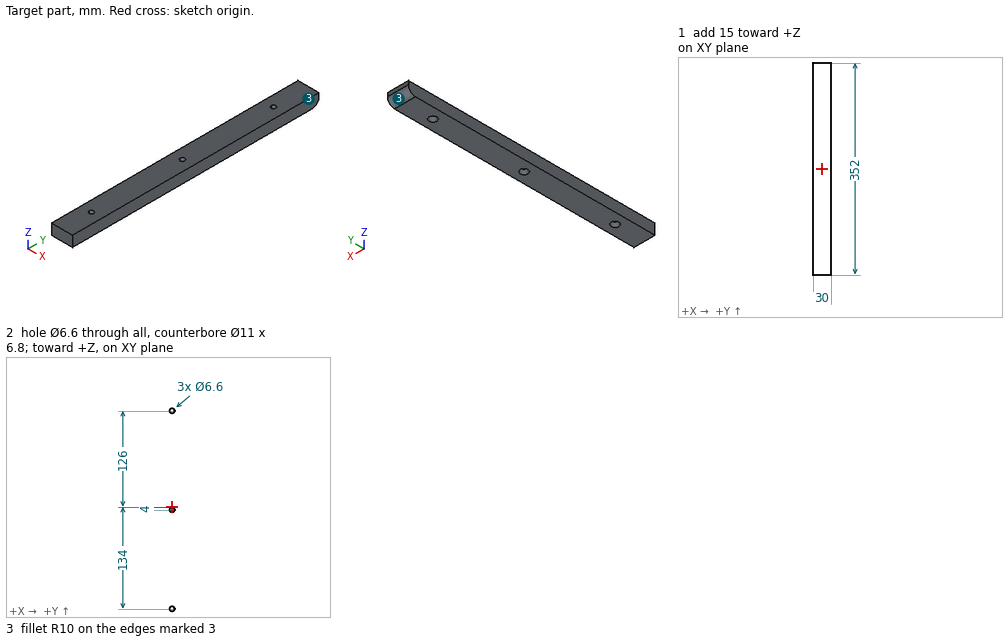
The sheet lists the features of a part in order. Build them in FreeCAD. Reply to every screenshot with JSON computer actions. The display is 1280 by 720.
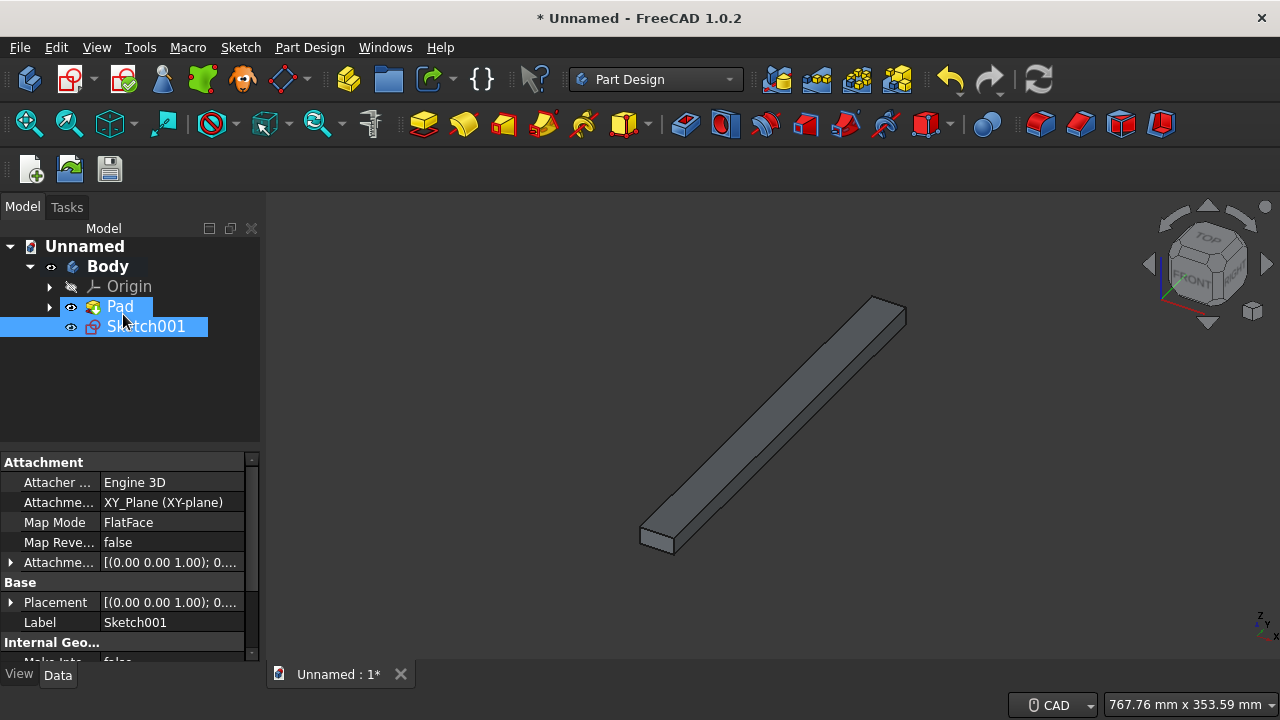
{"action": "left_click", "coordinate": [726, 124]}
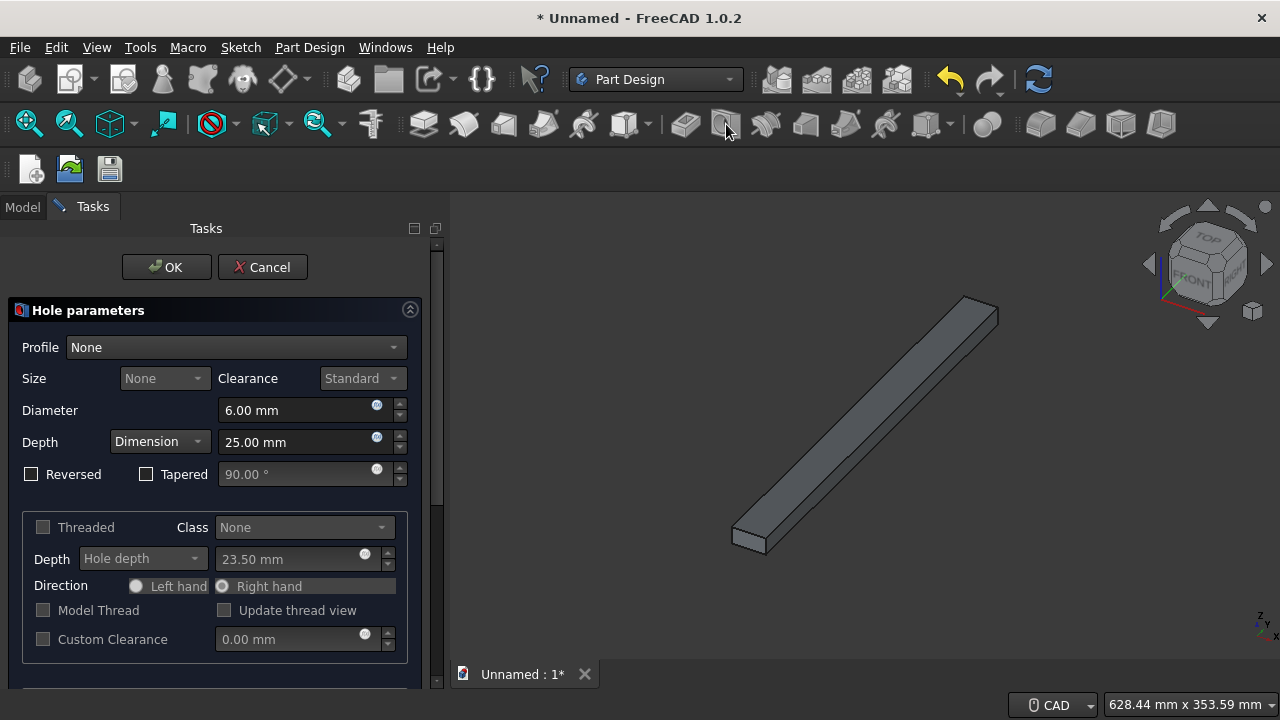
{"action": "triple_click", "coordinate": [305, 410]}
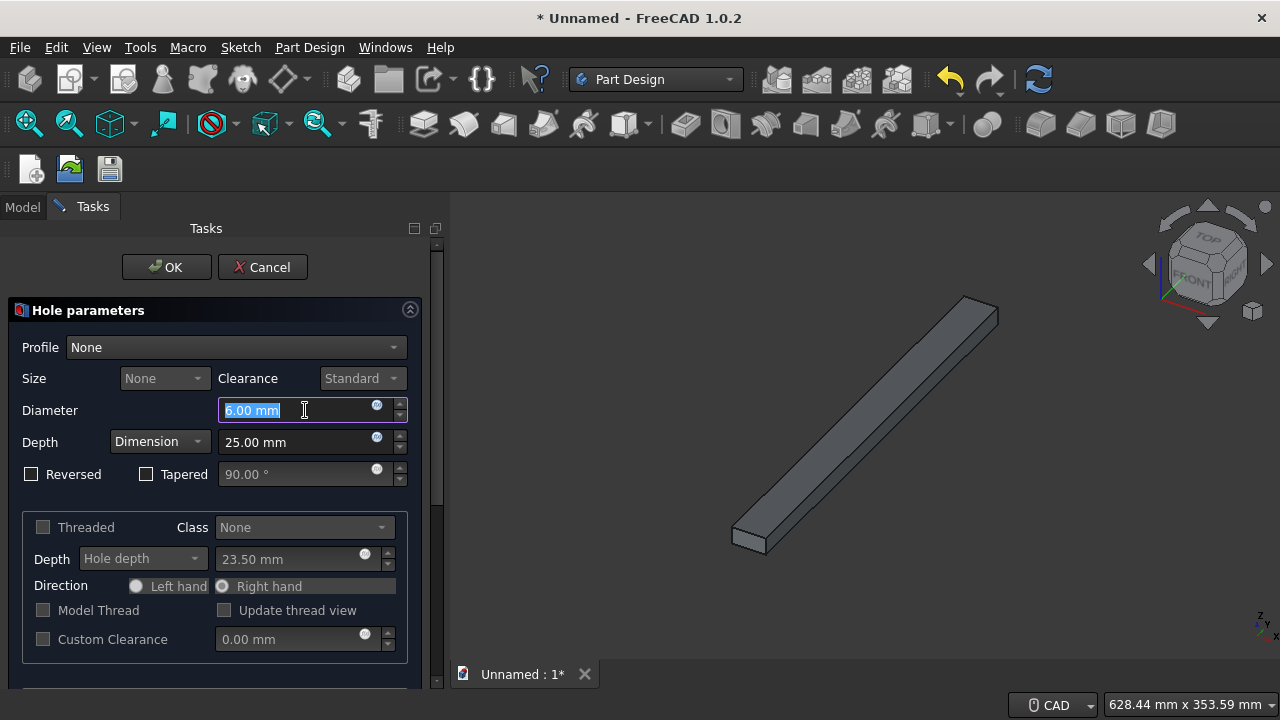
{"action": "type", "text": "6.6"}
{"action": "key", "text": "Tab"}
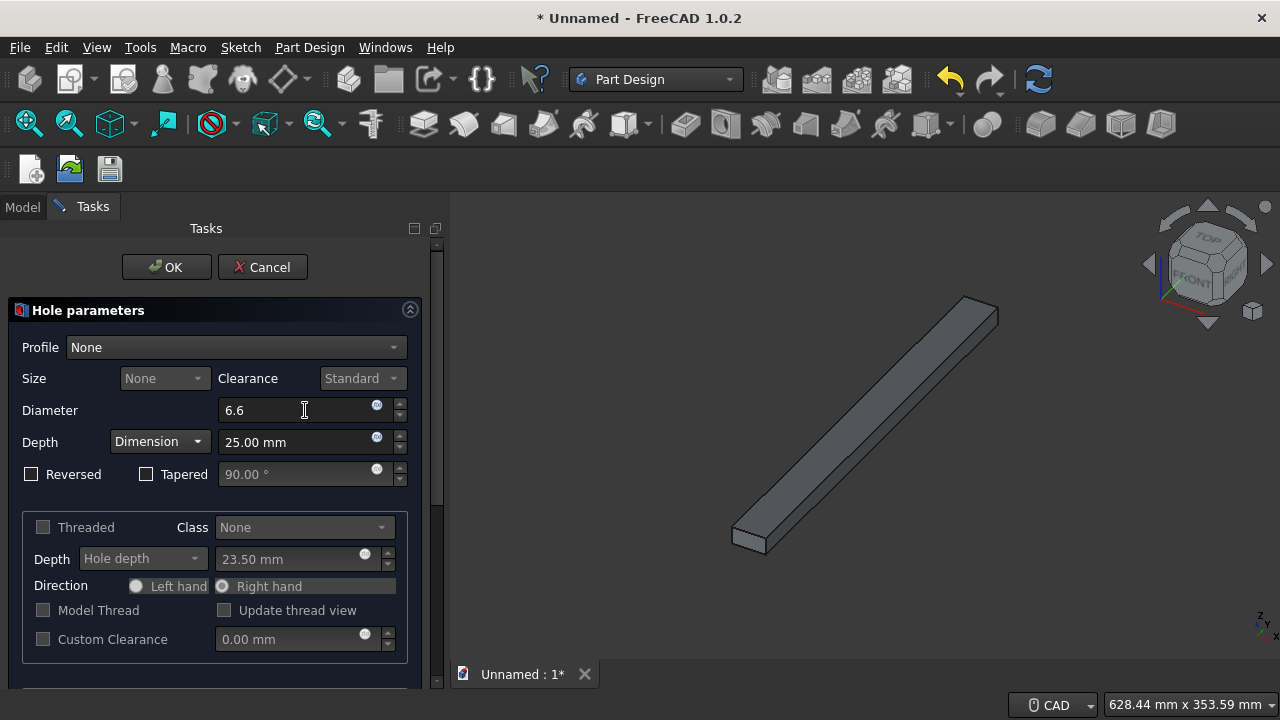
{"action": "left_click", "coordinate": [161, 442]}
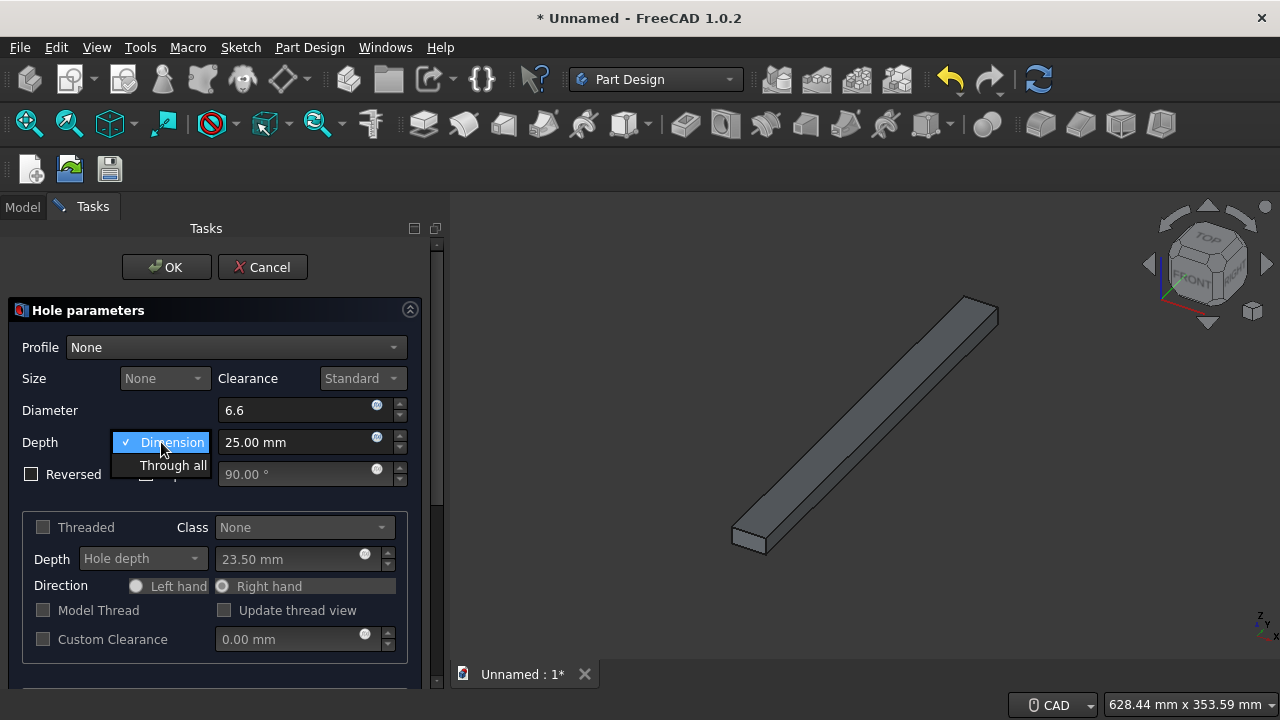
{"action": "left_click", "coordinate": [160, 466]}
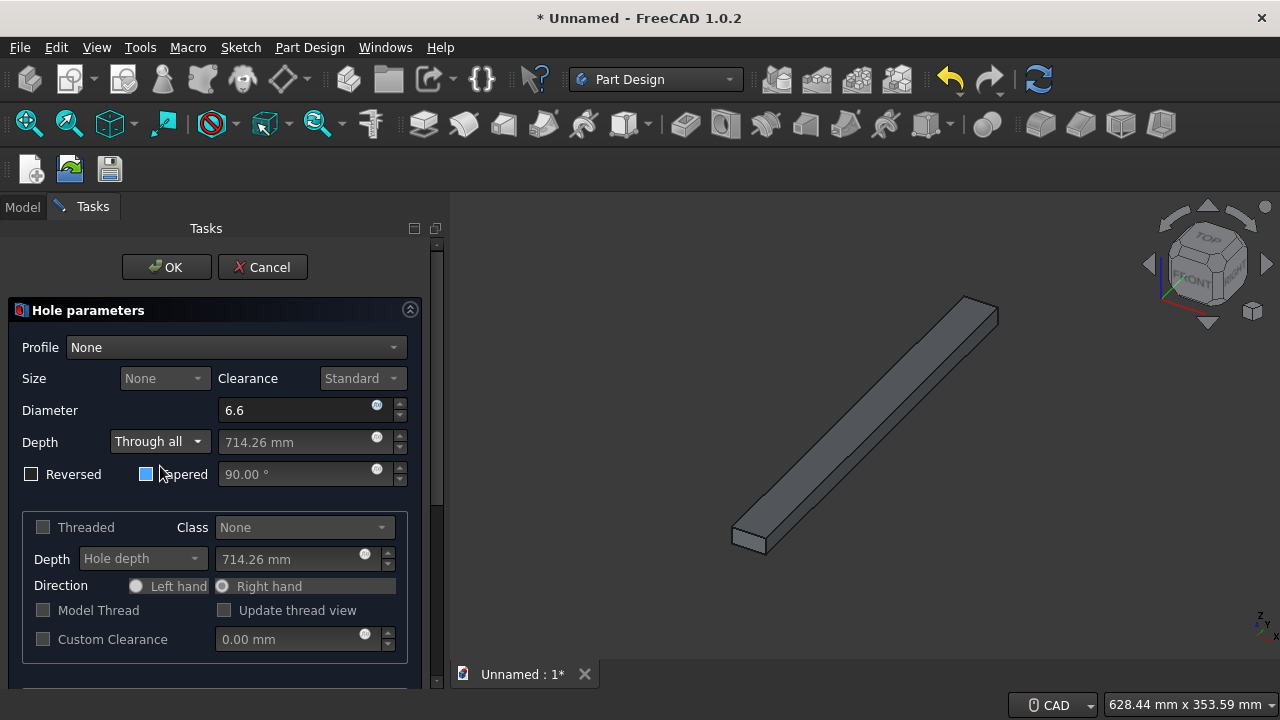
{"action": "left_click", "coordinate": [30, 474]}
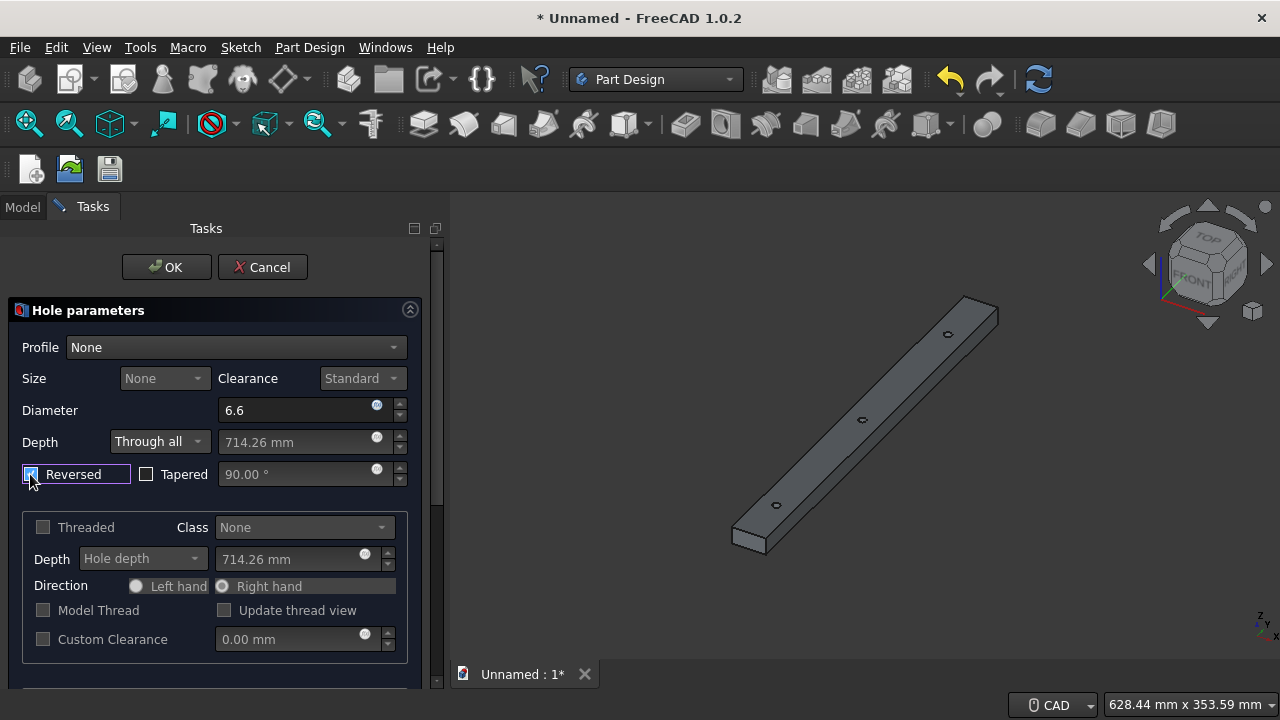
{"action": "scroll", "coordinate": [437, 463], "scroll_direction": "down", "scroll_amount": 2}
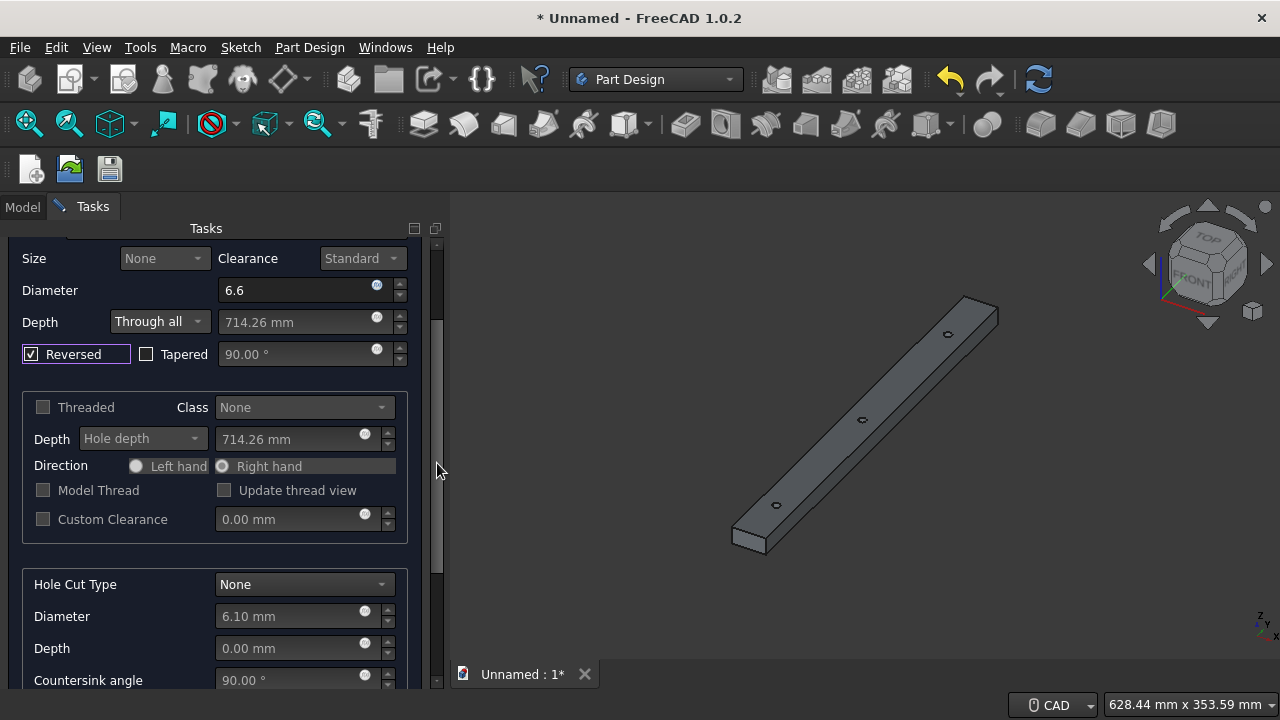
{"action": "left_click", "coordinate": [306, 584]}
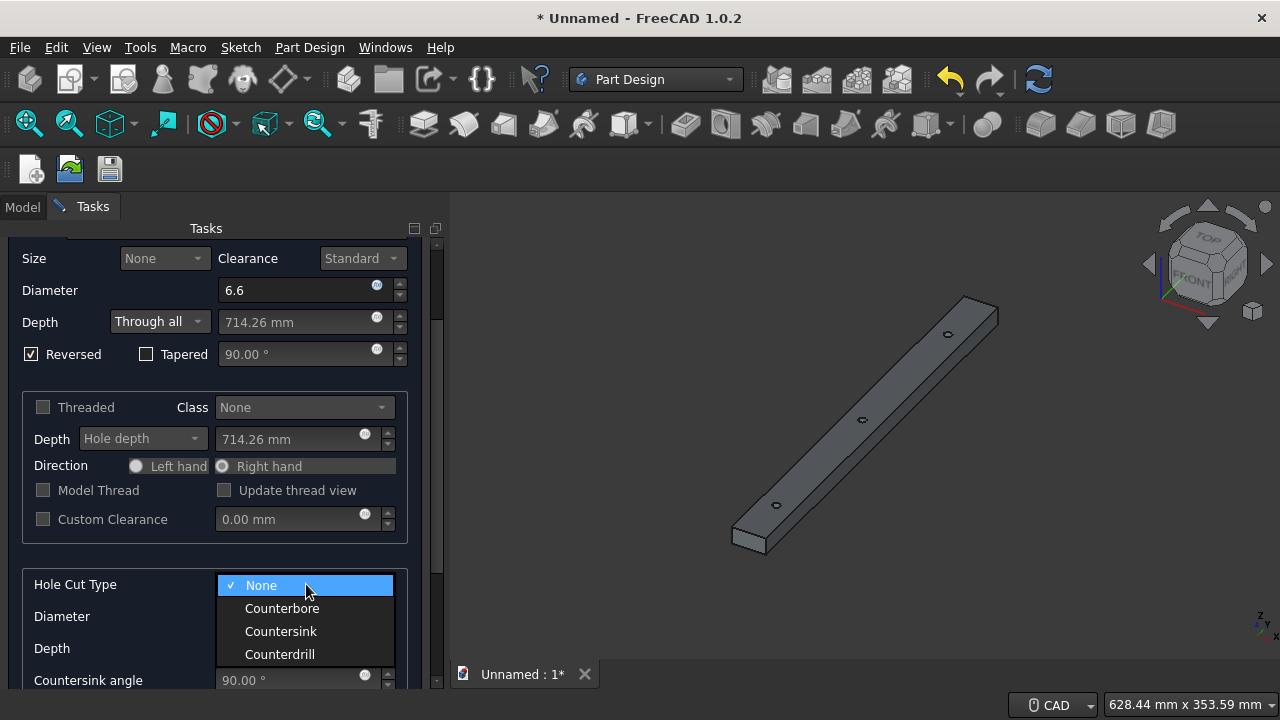
{"action": "left_click", "coordinate": [304, 608]}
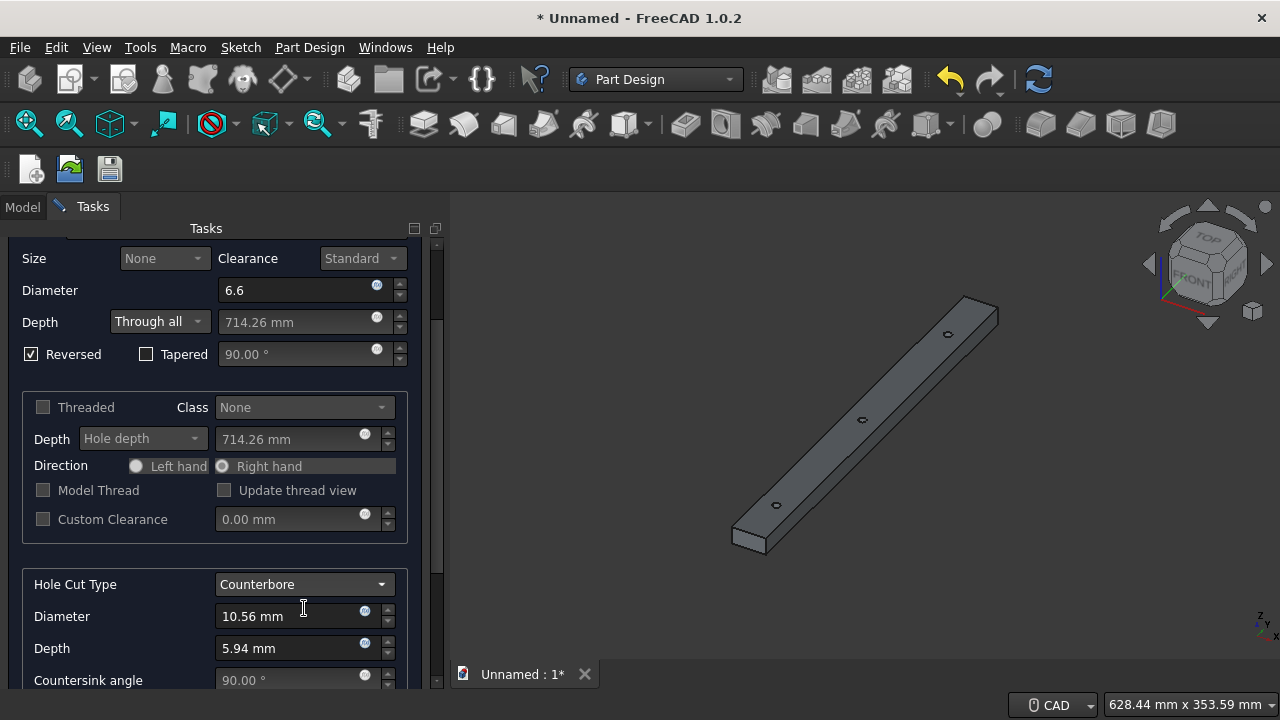
{"action": "triple_click", "coordinate": [298, 616]}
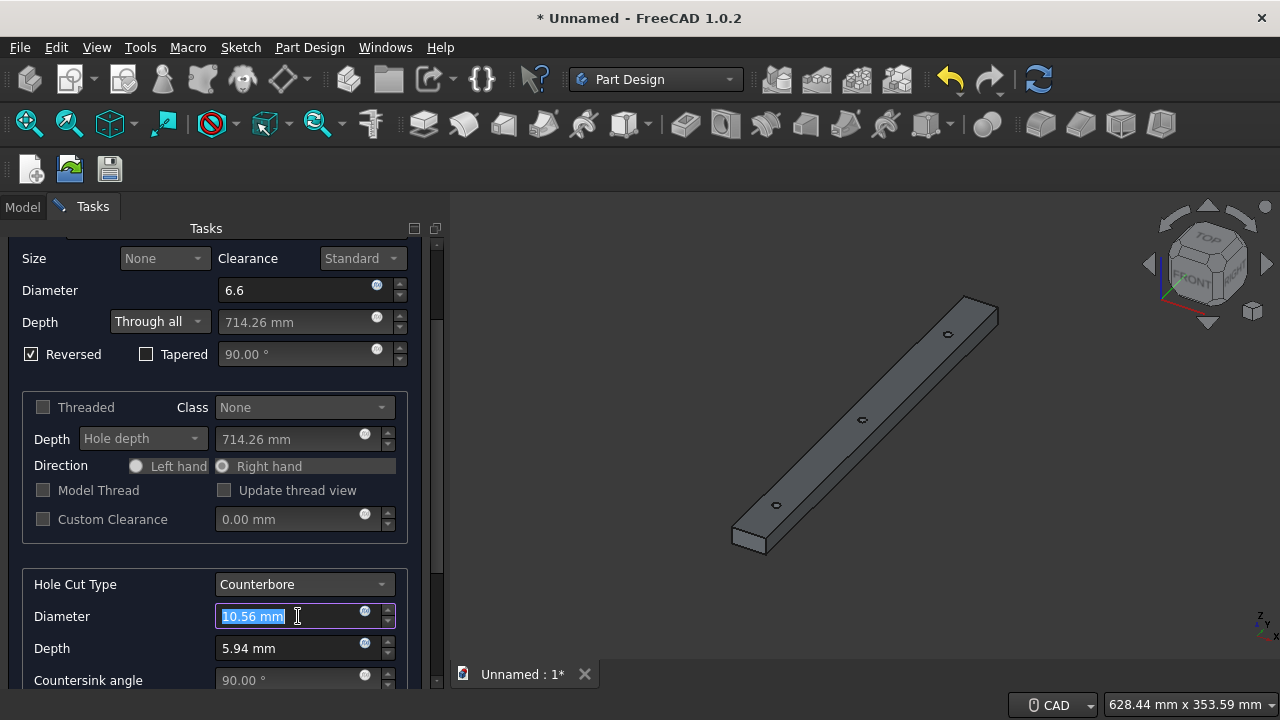
{"action": "type", "text": "11"}
{"action": "key", "text": "Tab"}